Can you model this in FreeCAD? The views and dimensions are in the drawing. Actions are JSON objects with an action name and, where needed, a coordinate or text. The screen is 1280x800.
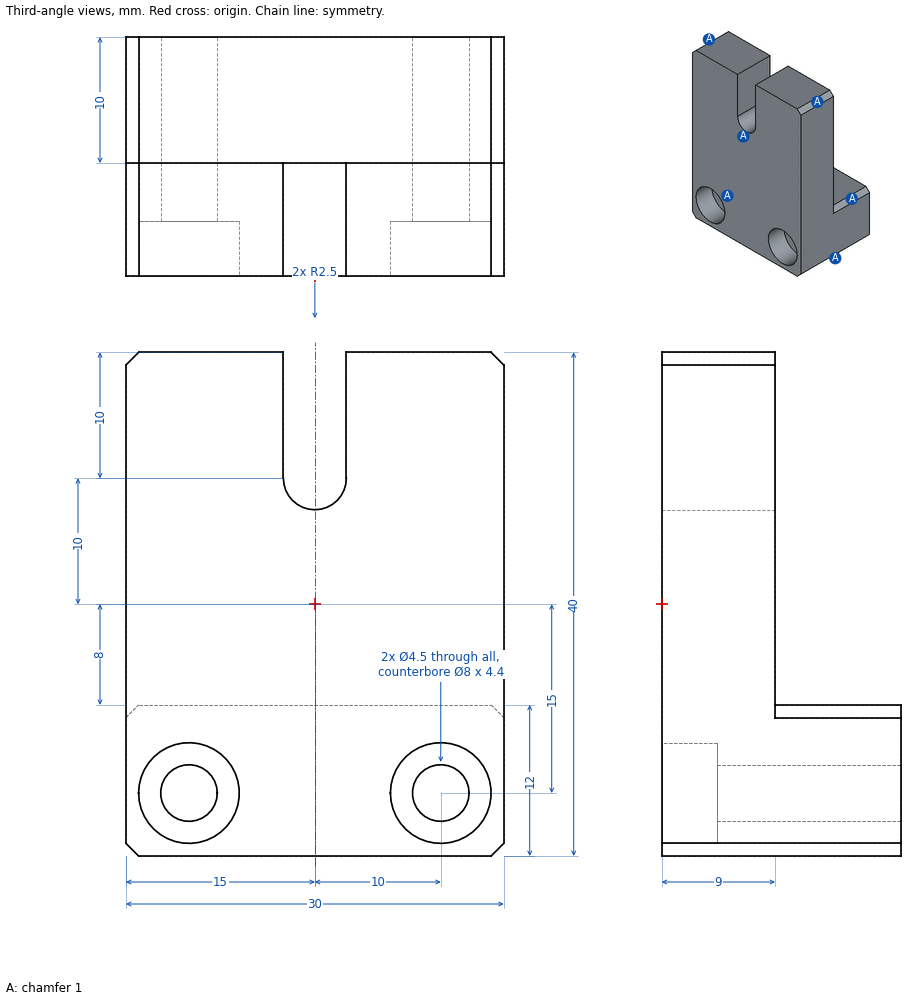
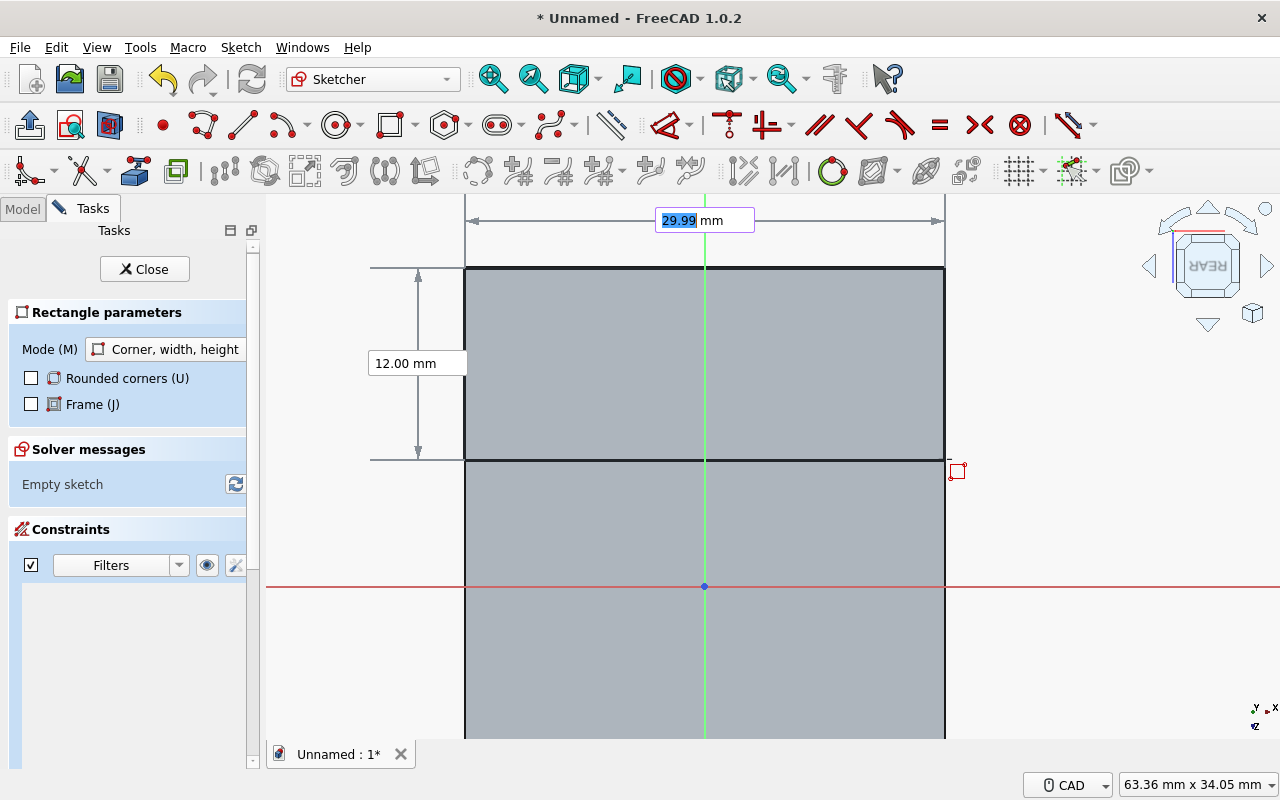
{"action": "type", "text": "30"}
{"action": "key", "text": "Tab"}
{"action": "type", "text": "12"}
{"action": "key", "text": "Return"}
{"action": "key", "text": "Escape"}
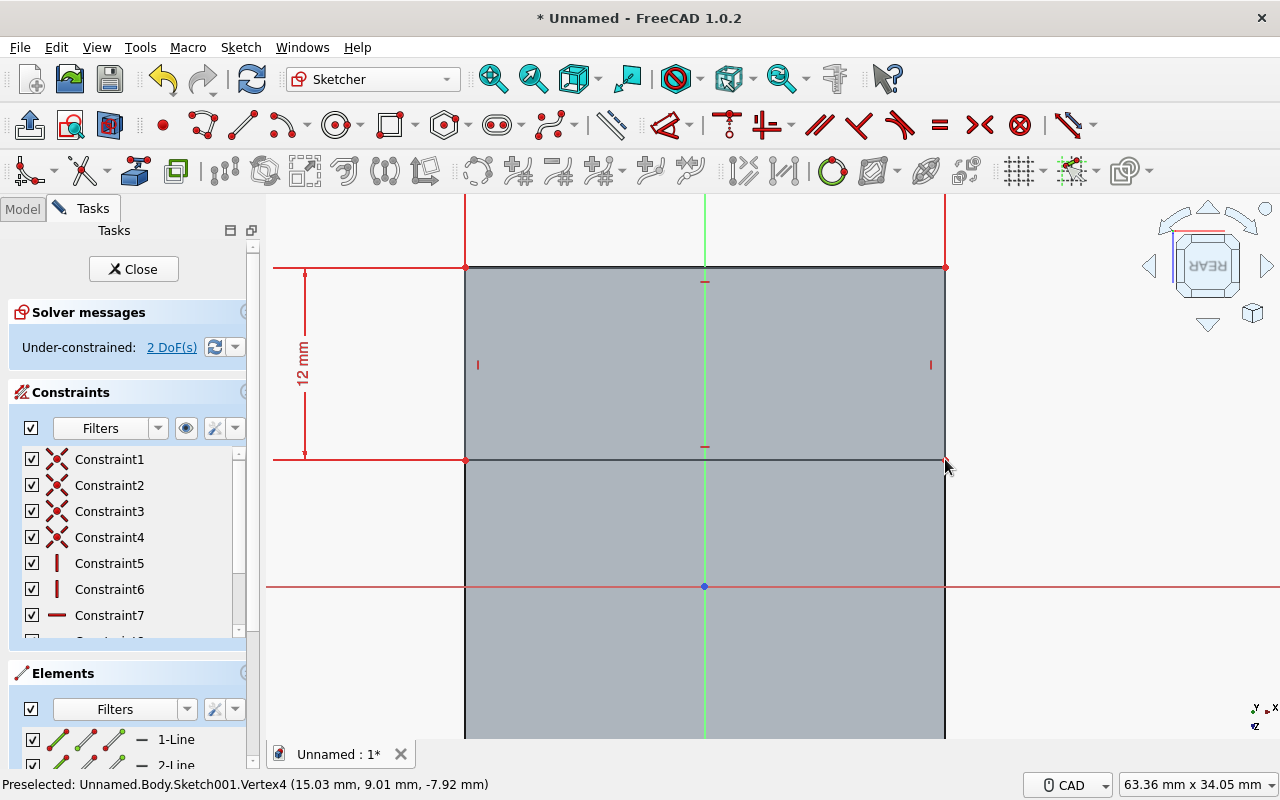
{"action": "left_click", "coordinate": [666, 126]}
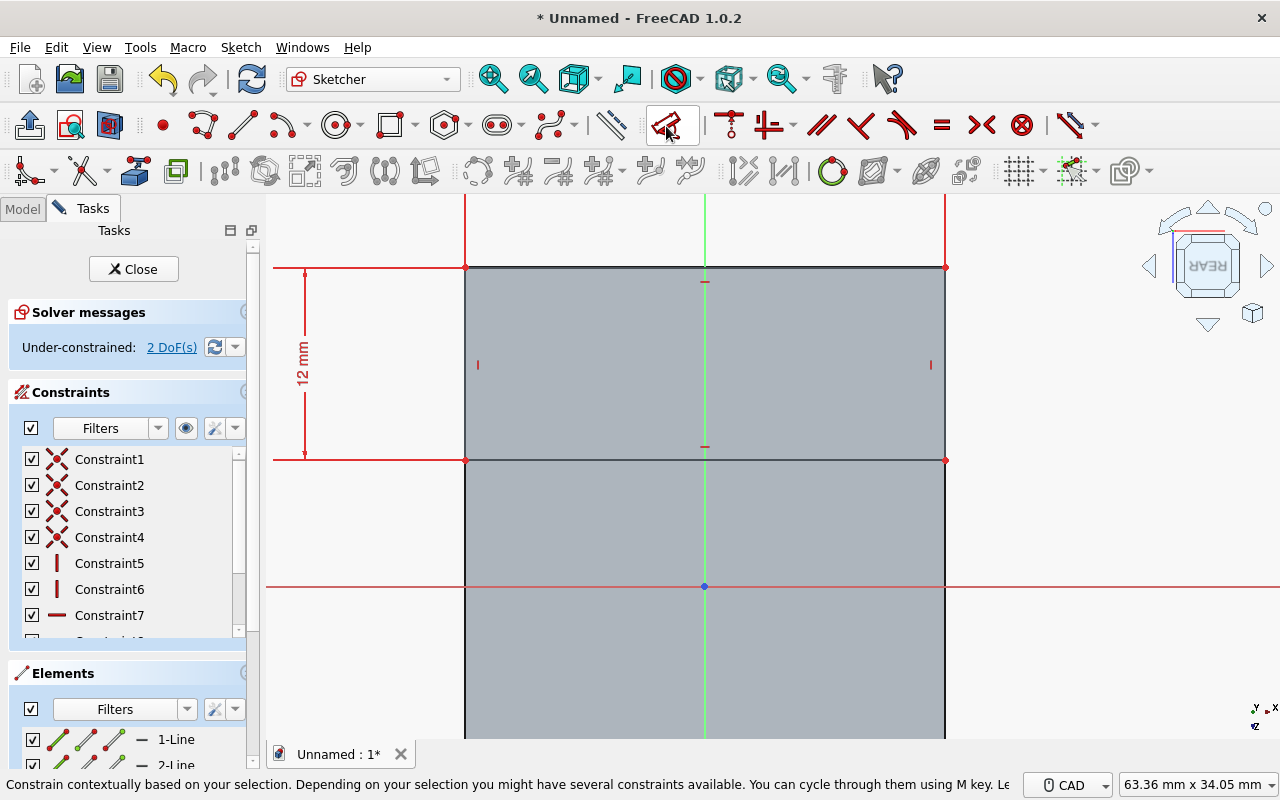
{"action": "left_click", "coordinate": [465, 460]}
{"action": "left_click", "coordinate": [431, 523]}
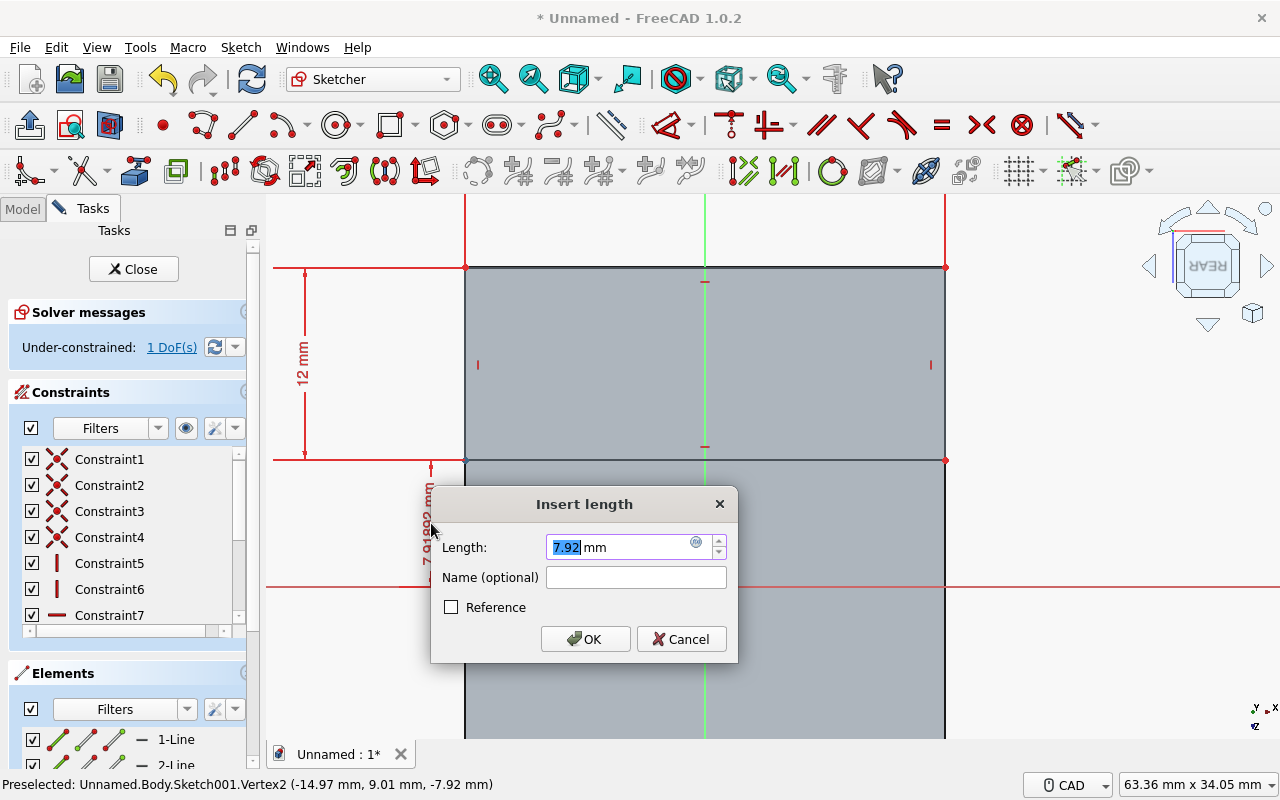
{"action": "type", "text": "8"}
{"action": "key", "text": "Return"}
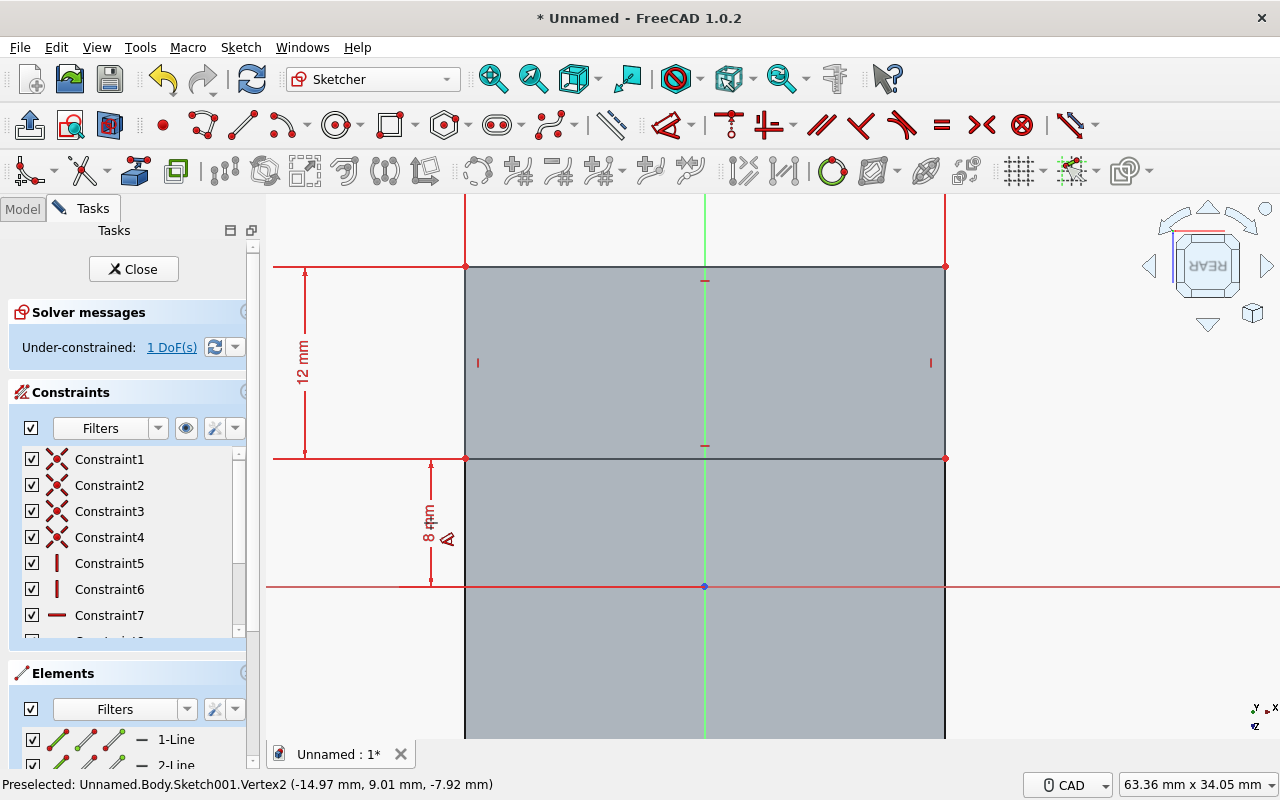
{"action": "left_click", "coordinate": [465, 267]}
{"action": "left_click", "coordinate": [585, 621]}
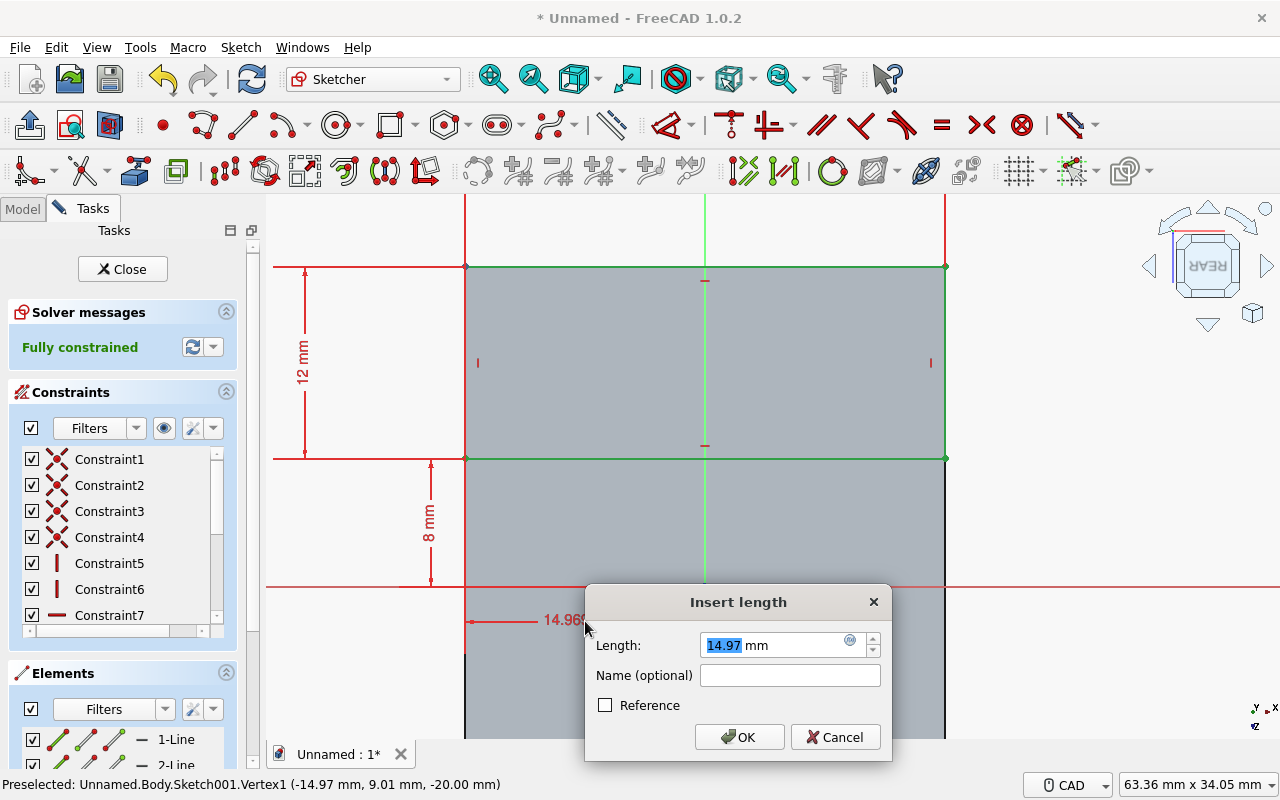
{"action": "type", "text": "15"}
{"action": "key", "text": "Return"}
{"action": "key", "text": "Escape"}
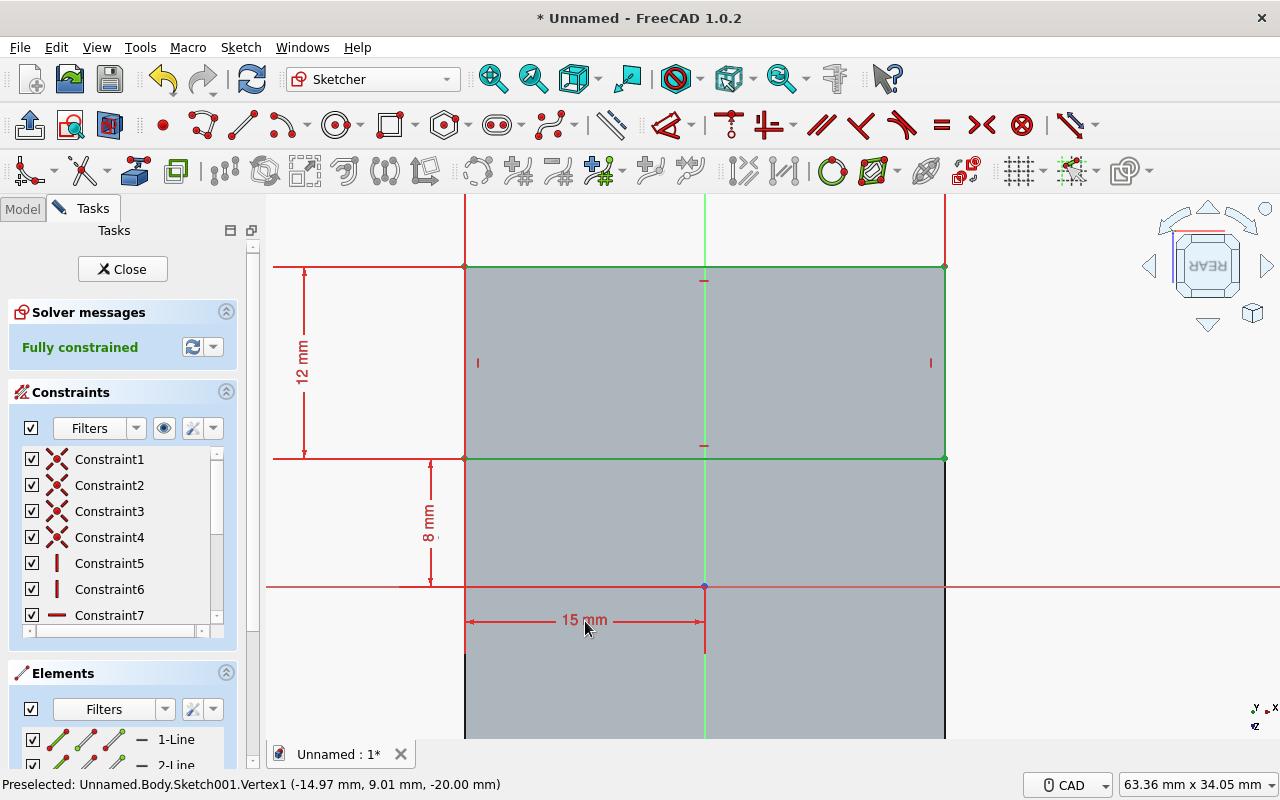
{"action": "left_click", "coordinate": [123, 269]}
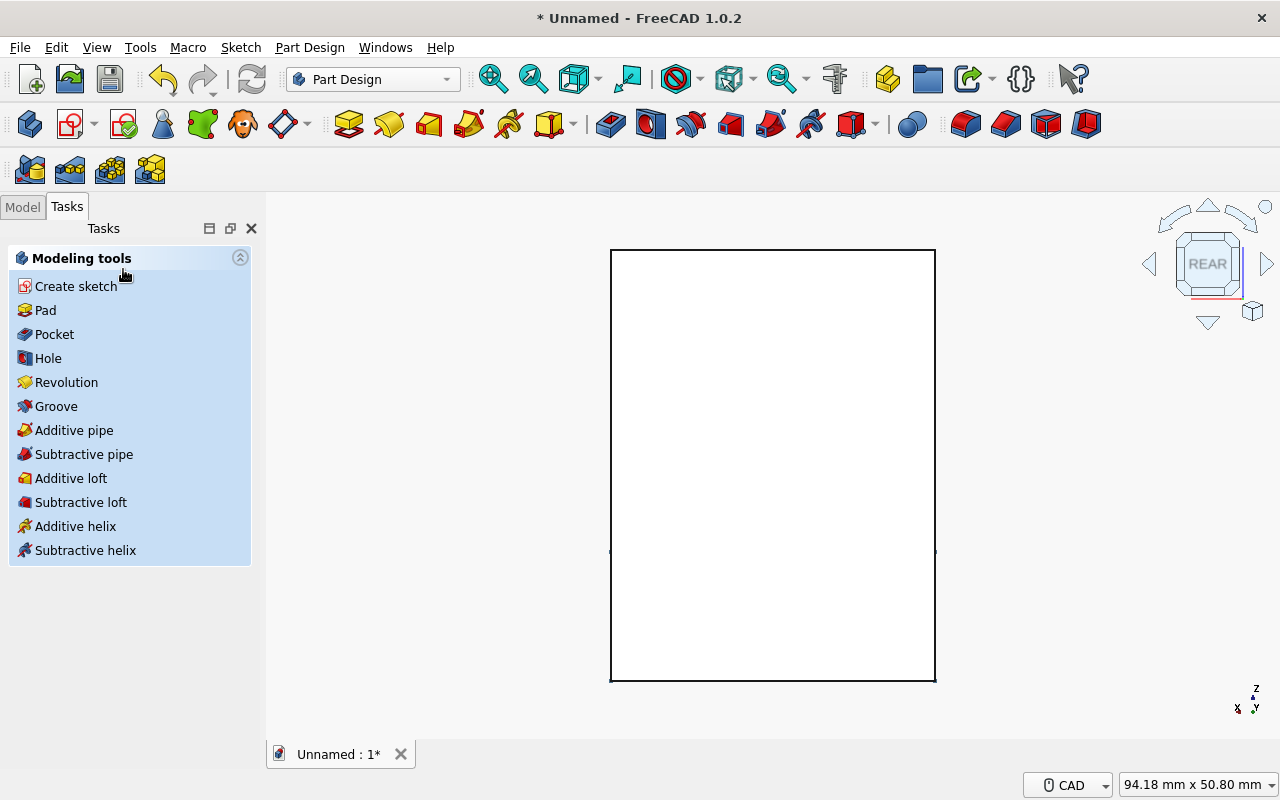
{"action": "left_click", "coordinate": [350, 124]}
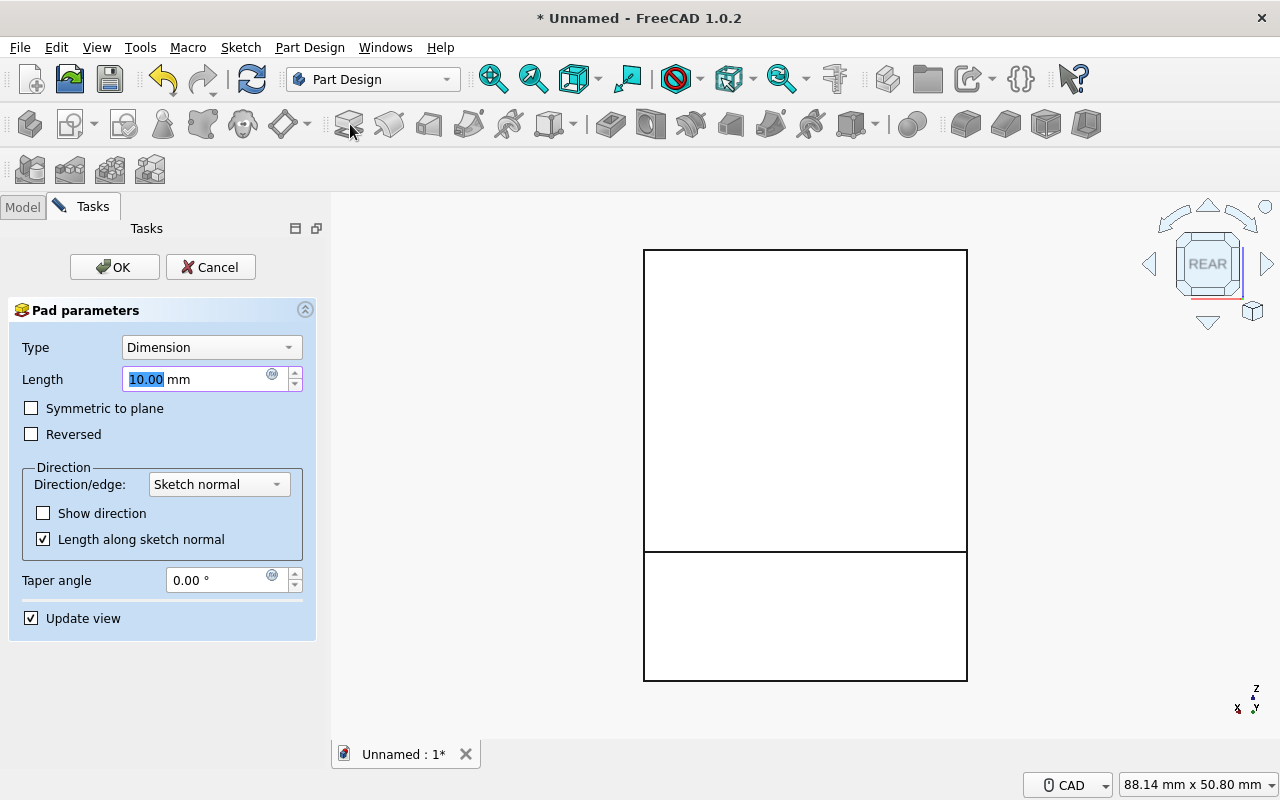
{"action": "type", "text": "10"}
{"action": "key", "text": "Tab"}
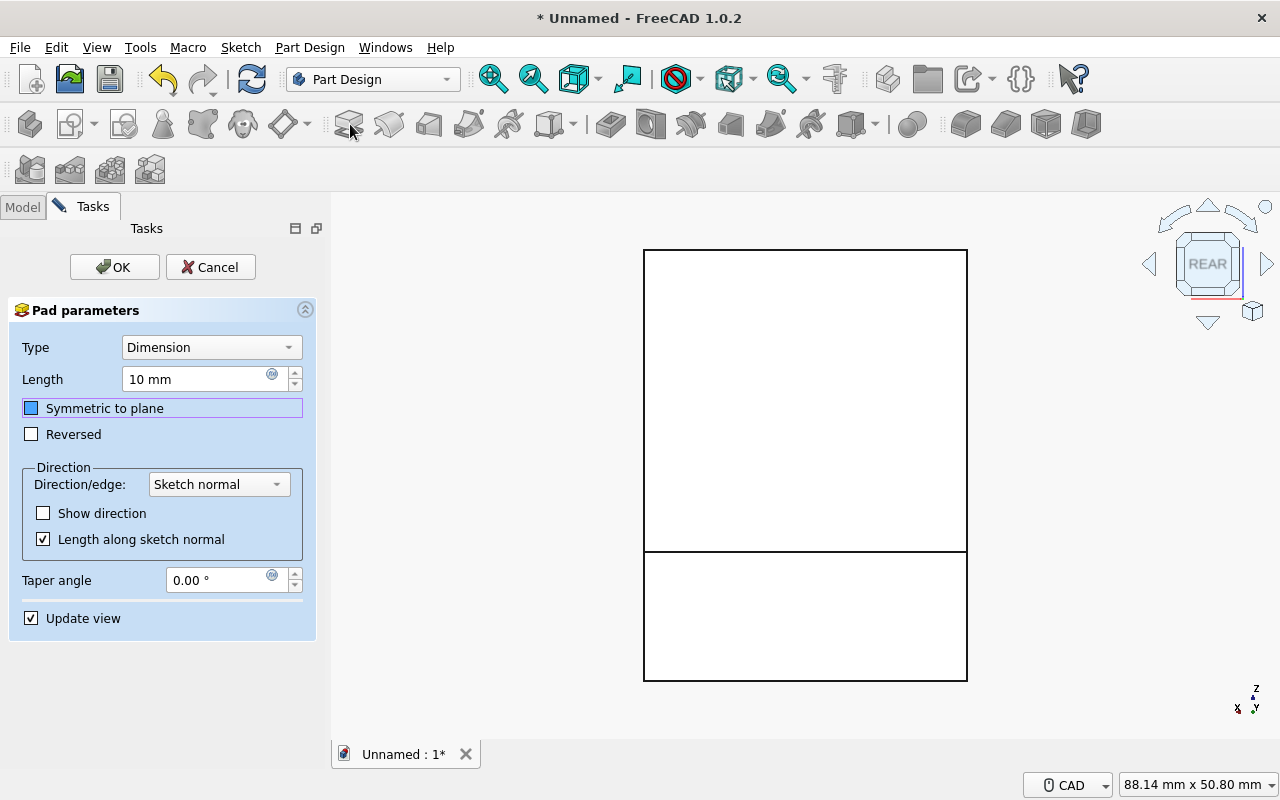
{"action": "left_click", "coordinate": [115, 267]}